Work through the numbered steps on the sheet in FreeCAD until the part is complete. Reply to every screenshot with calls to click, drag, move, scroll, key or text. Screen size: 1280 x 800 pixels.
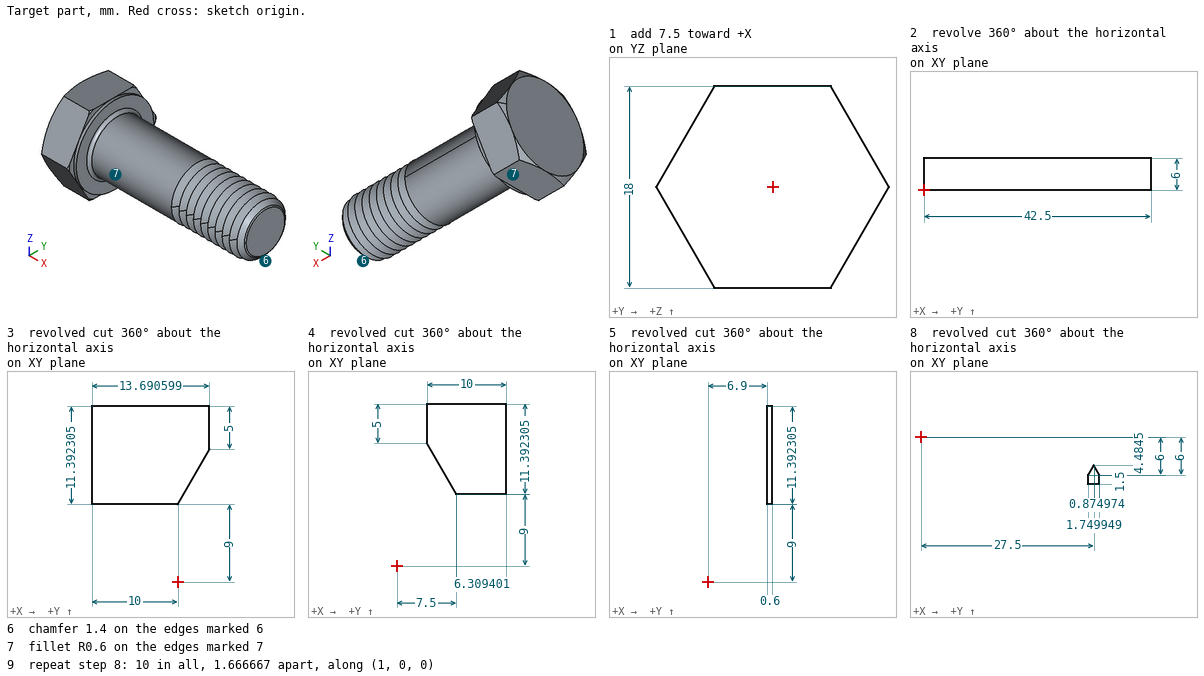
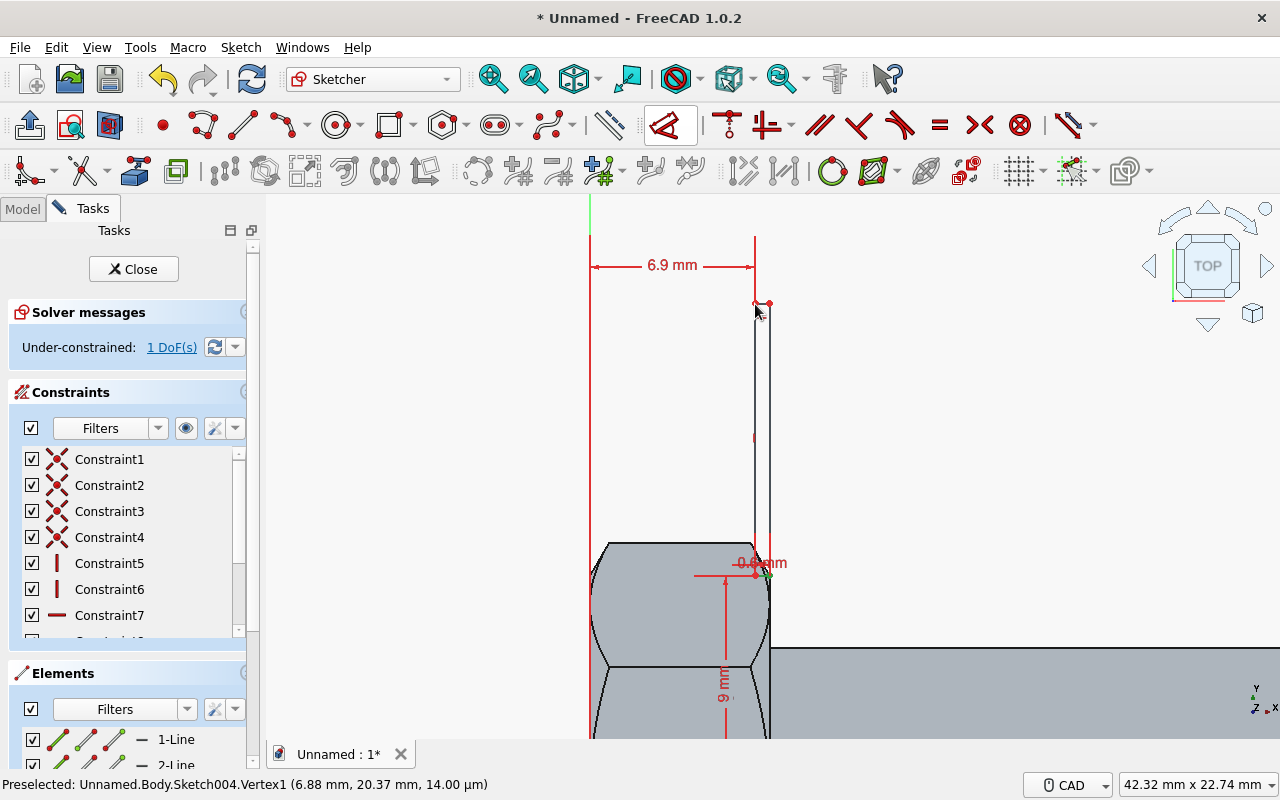
click(755, 385)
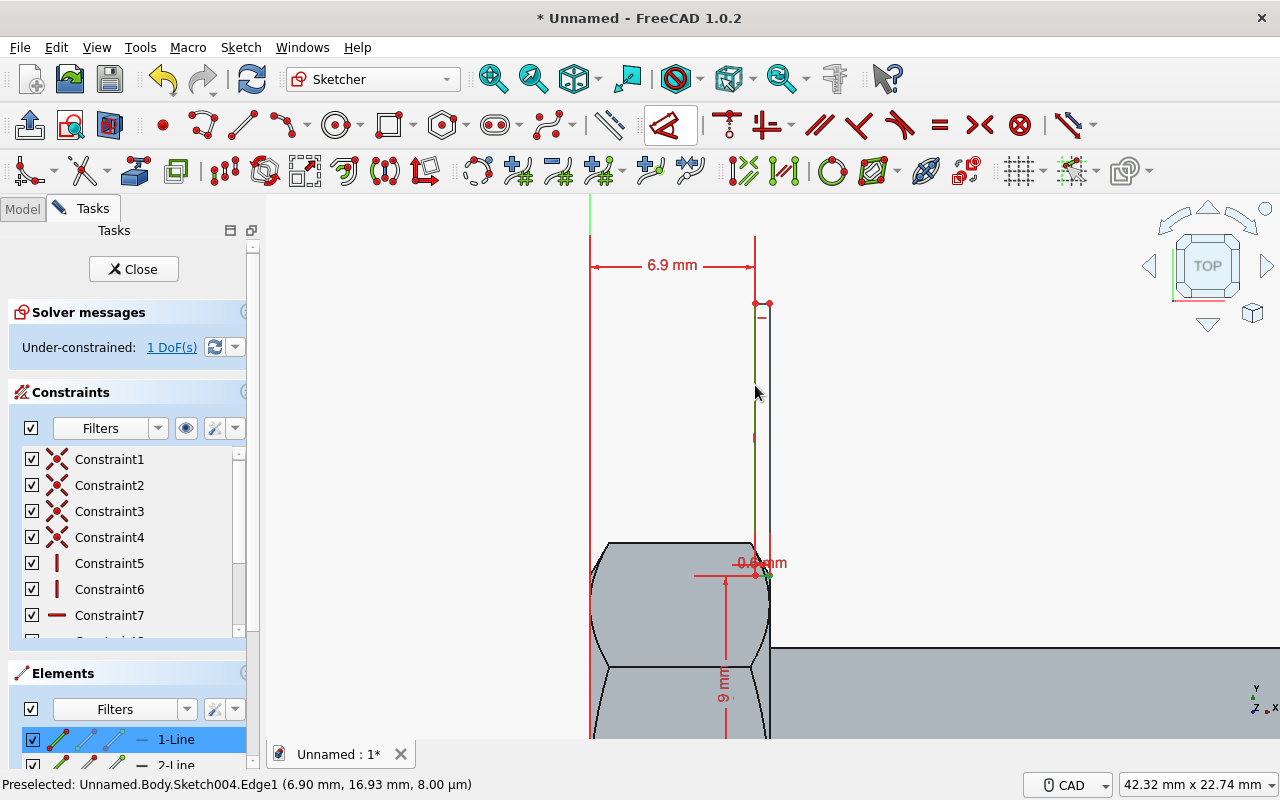
key(i)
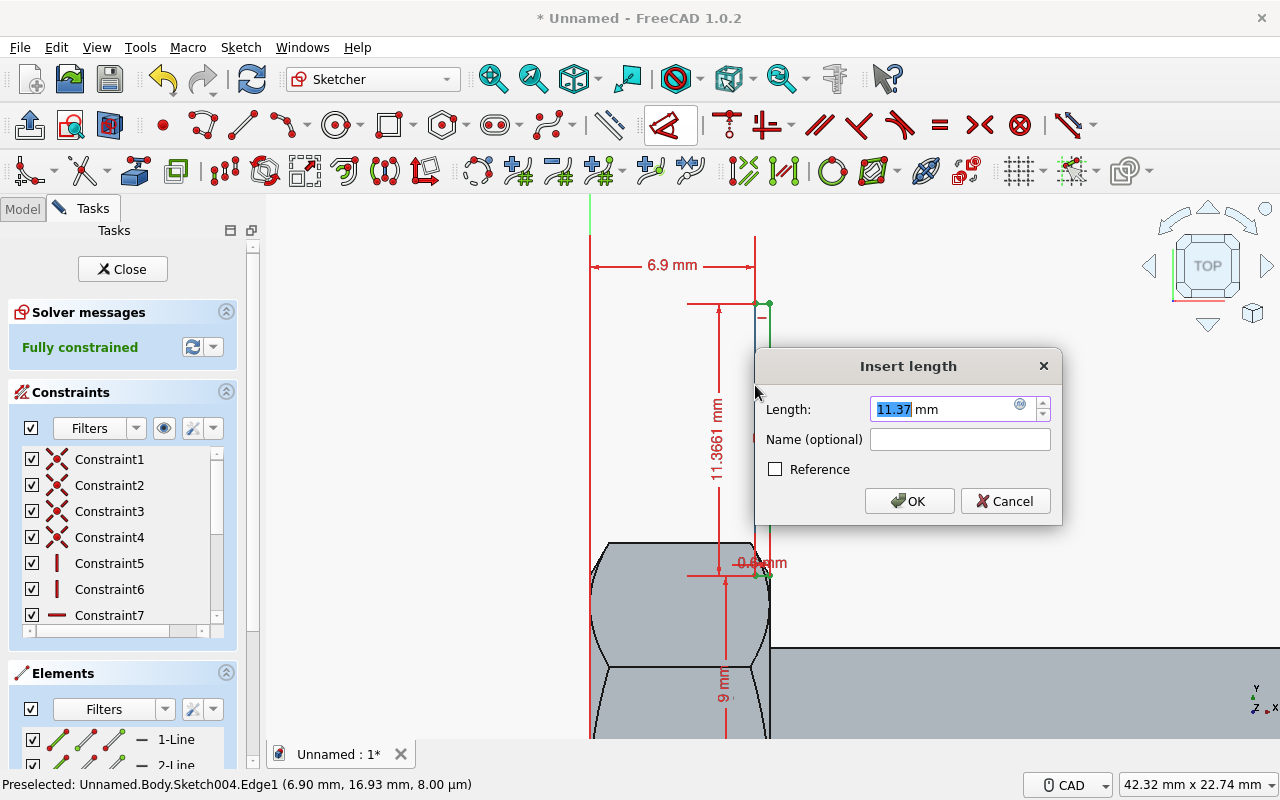
text(11.392305)
key(Return)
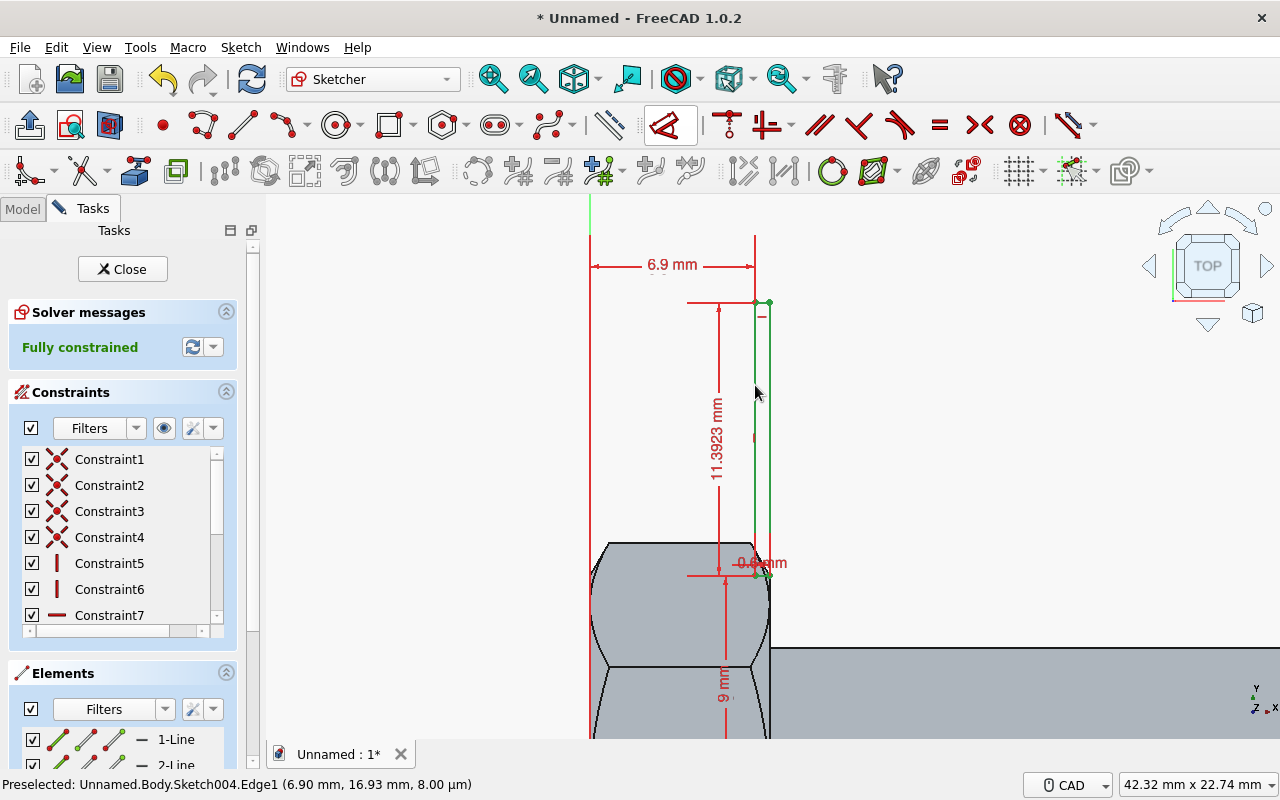
click(123, 269)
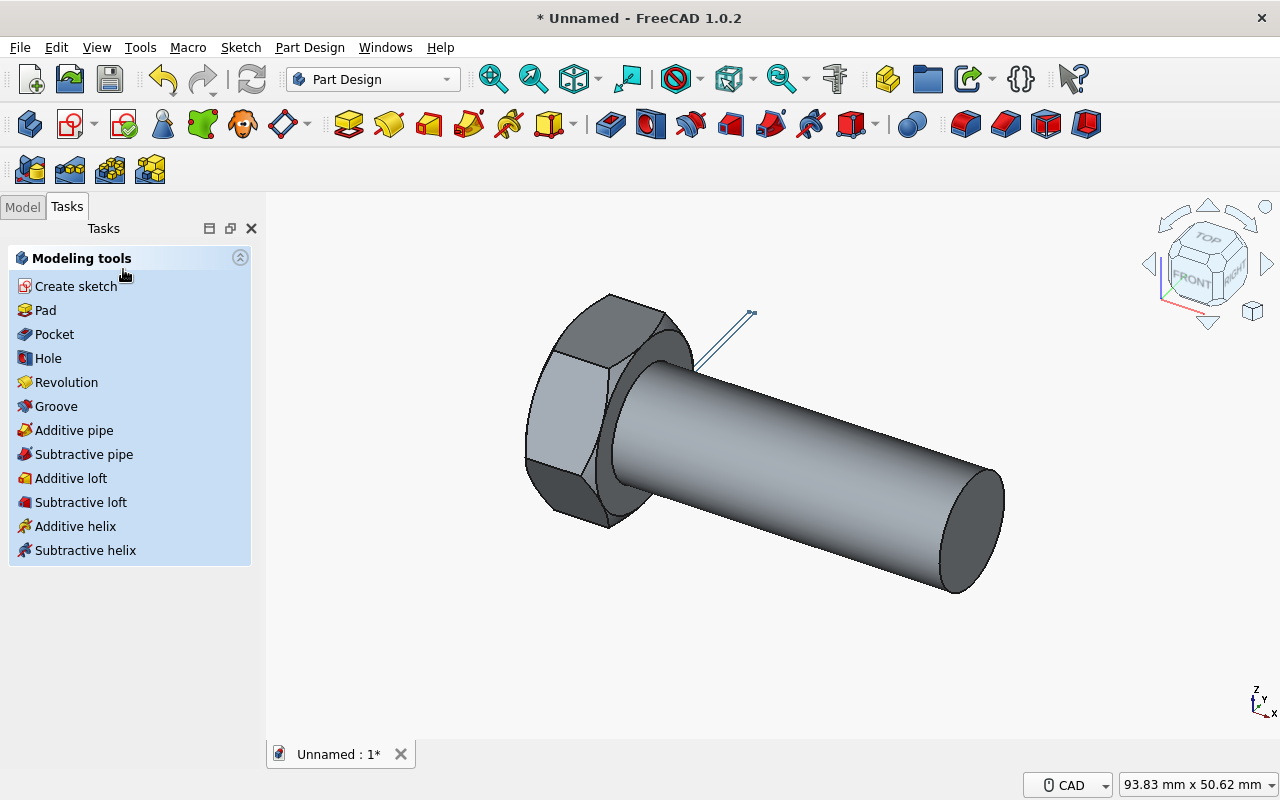
click(692, 124)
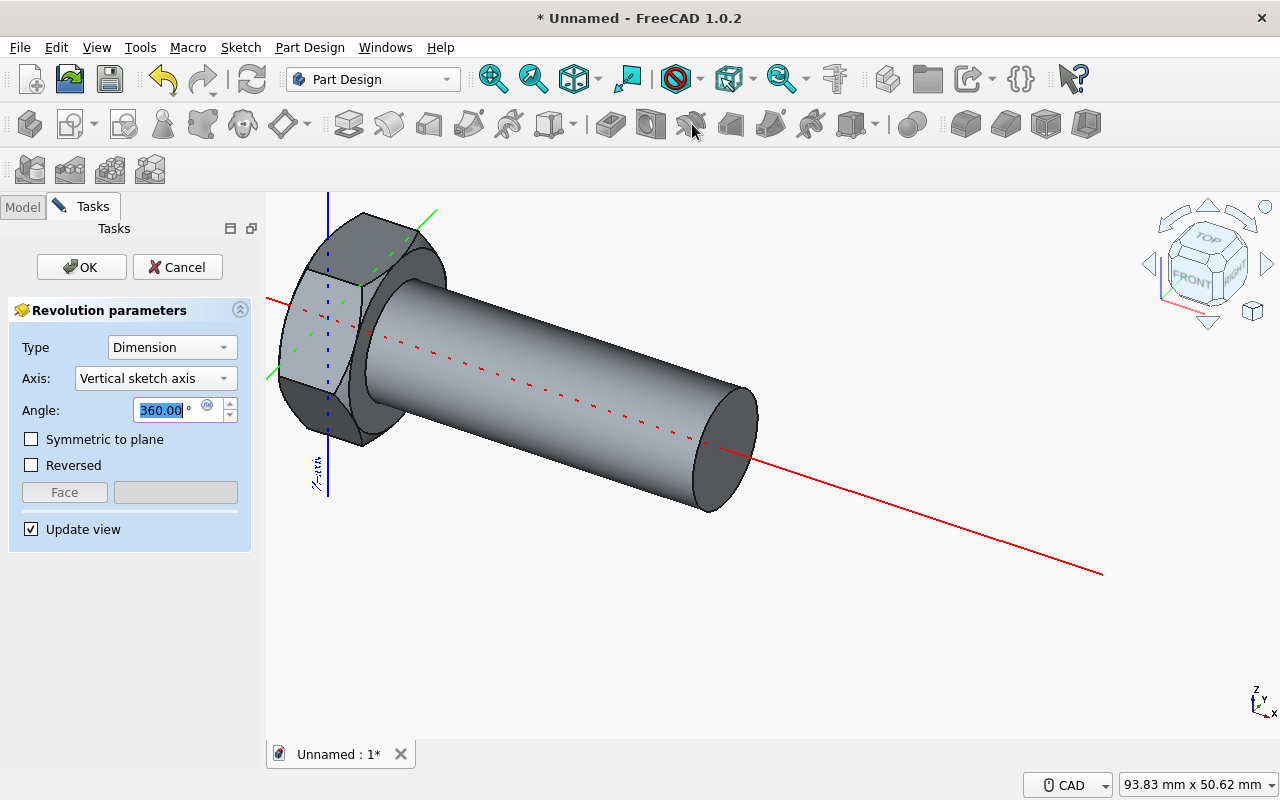
click(156, 378)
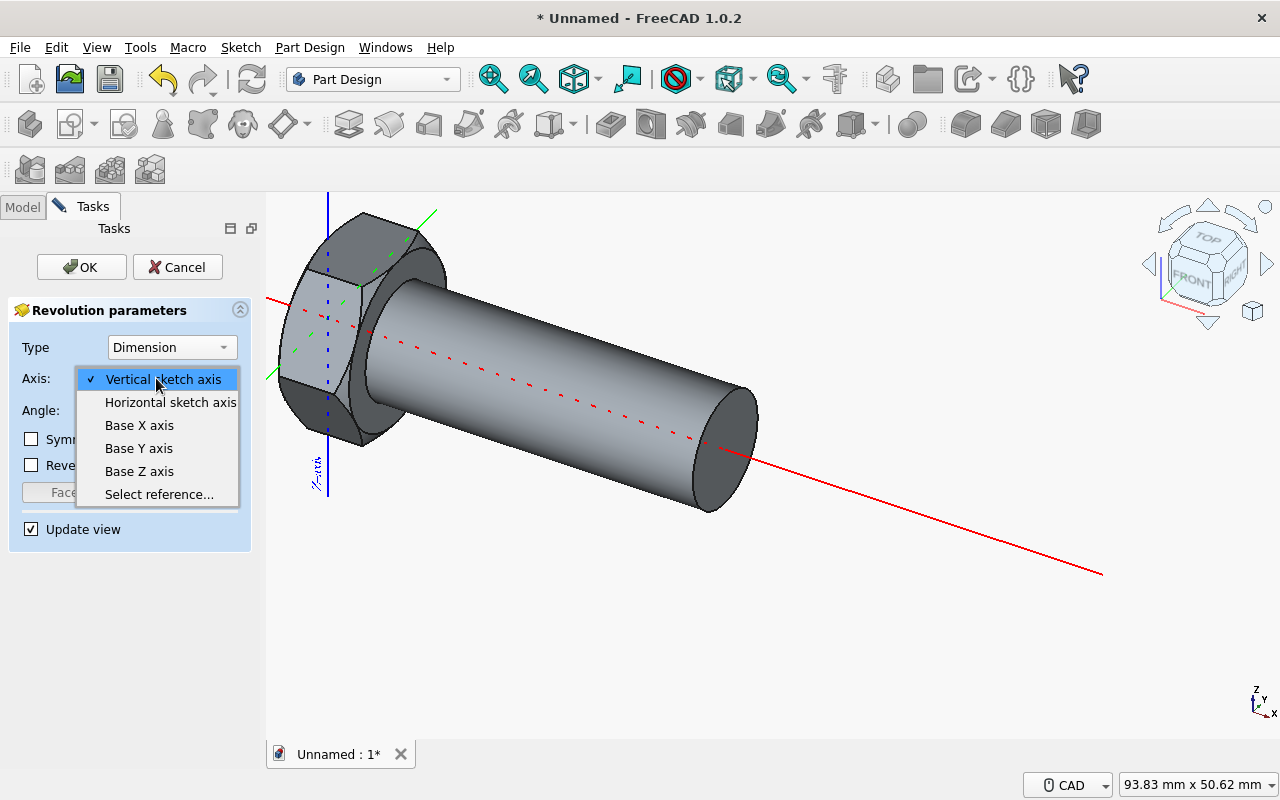
click(156, 402)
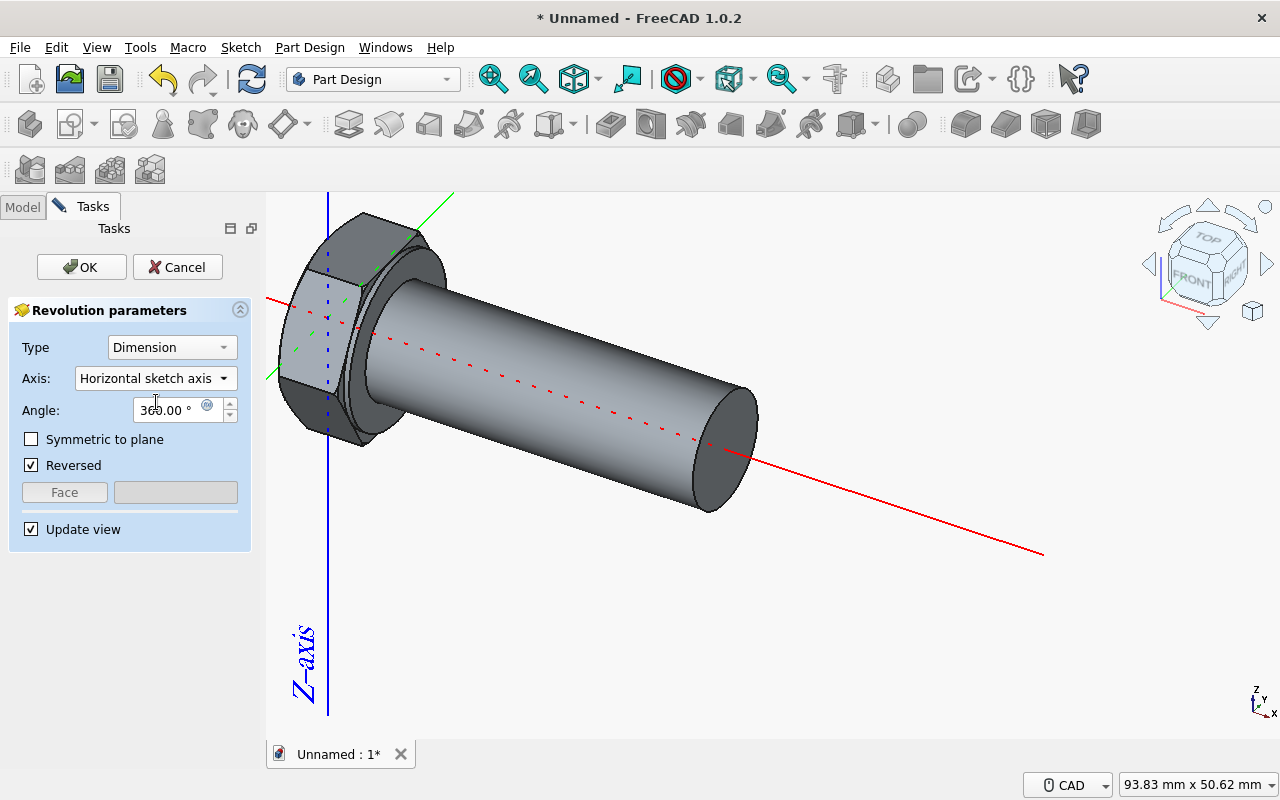
click(82, 267)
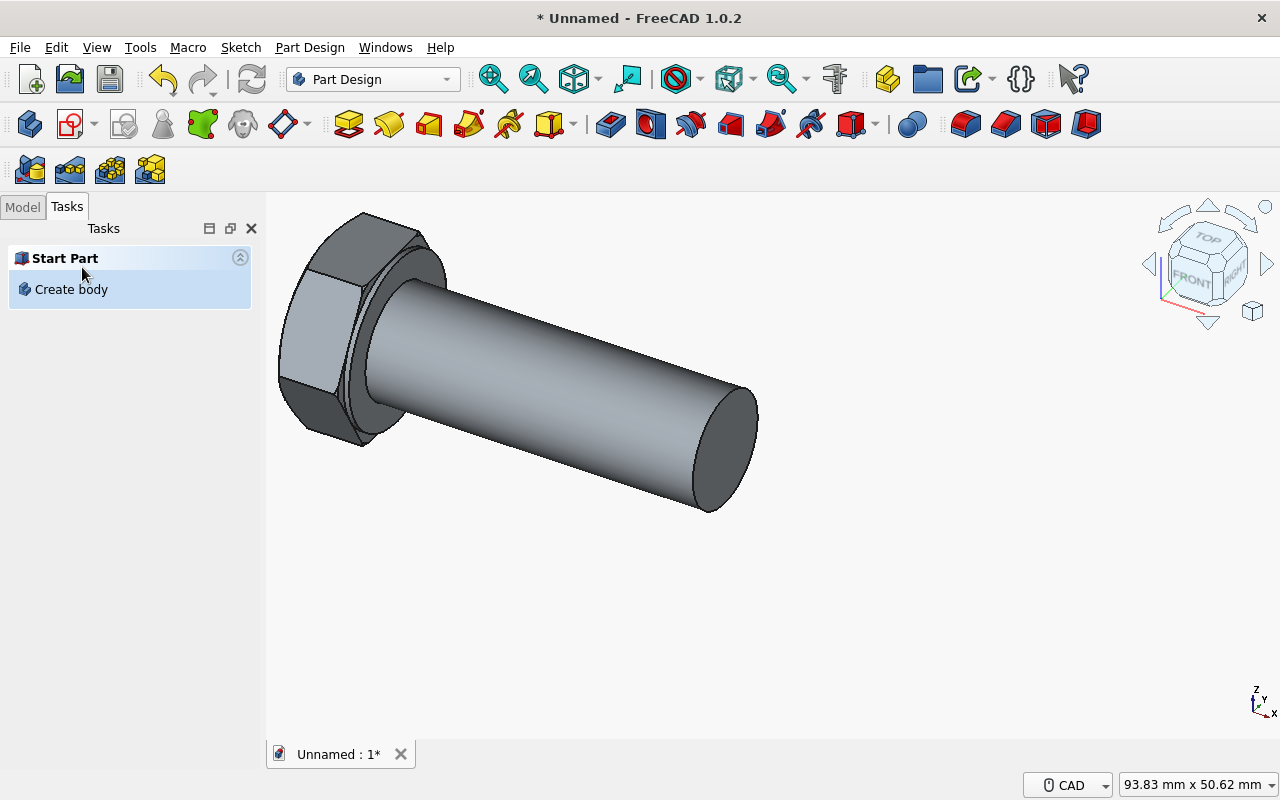
key(v)
key(f)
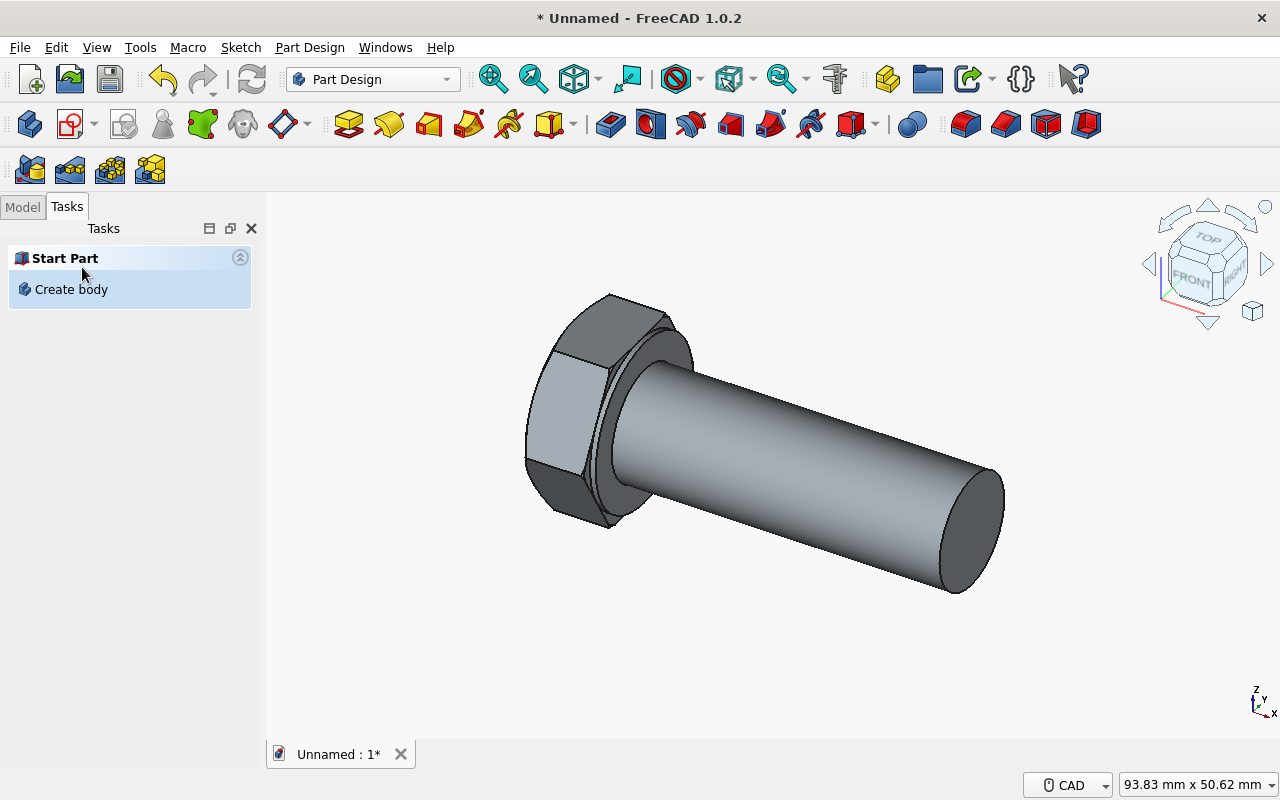
click(939, 563)